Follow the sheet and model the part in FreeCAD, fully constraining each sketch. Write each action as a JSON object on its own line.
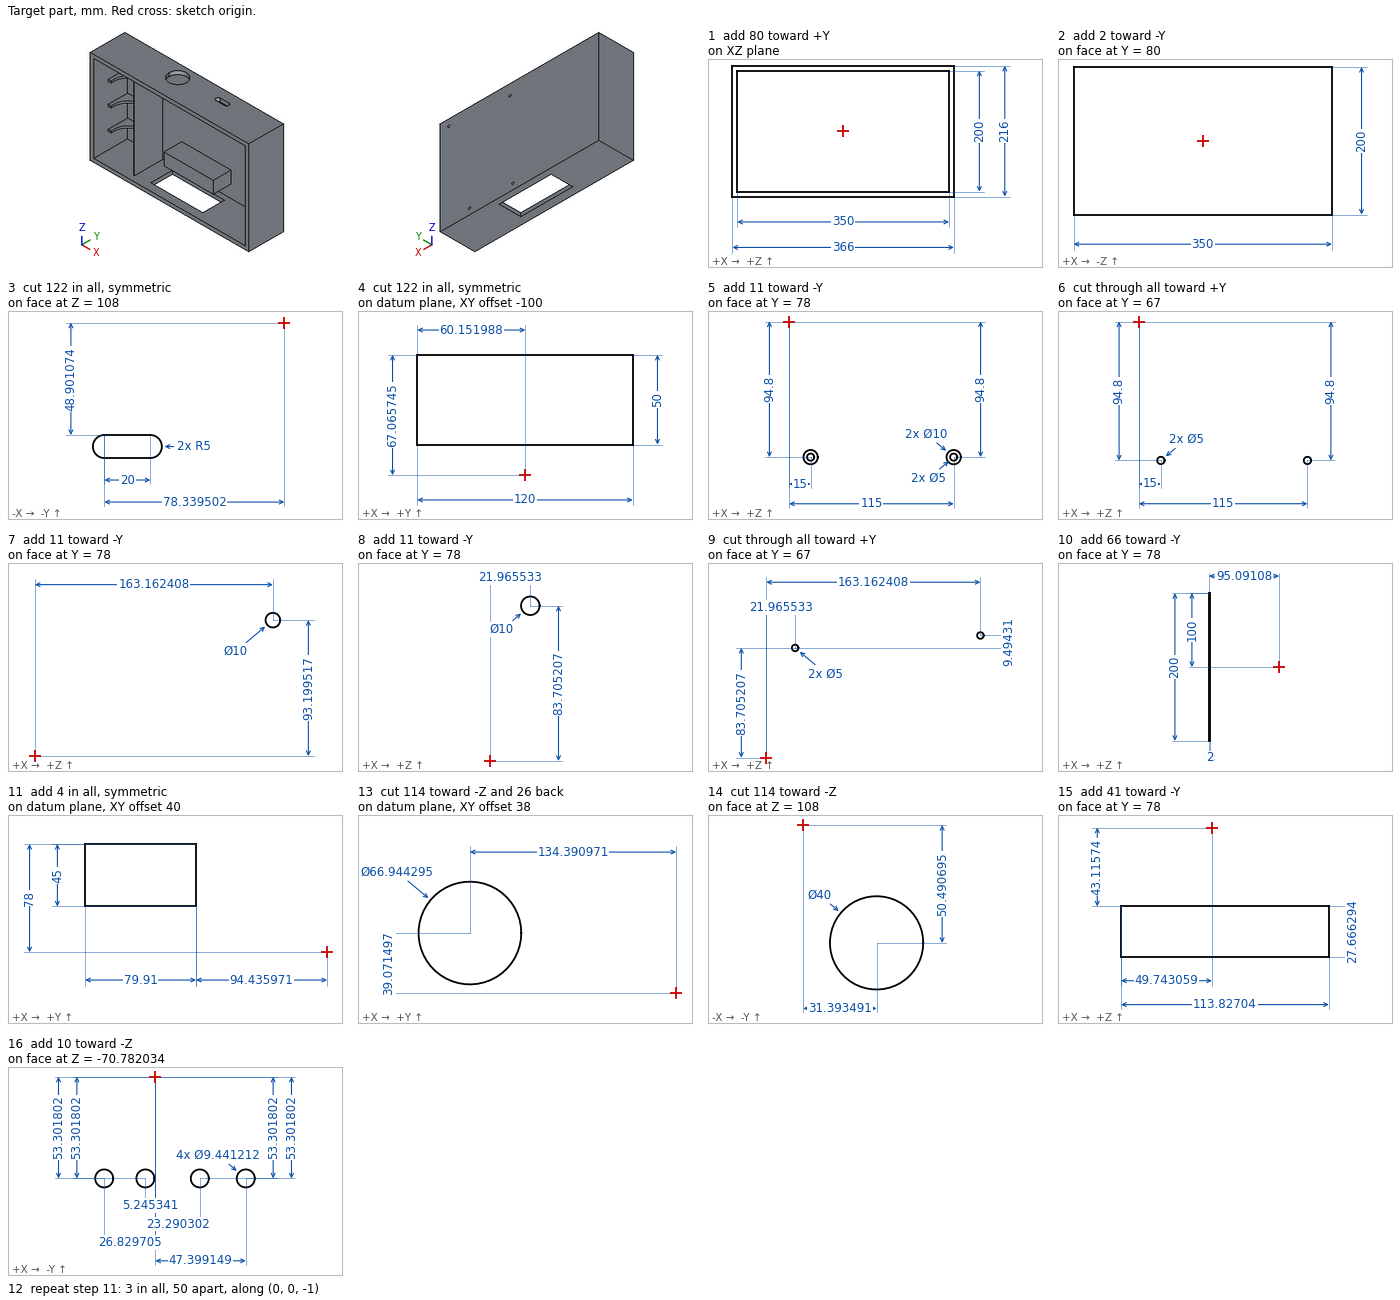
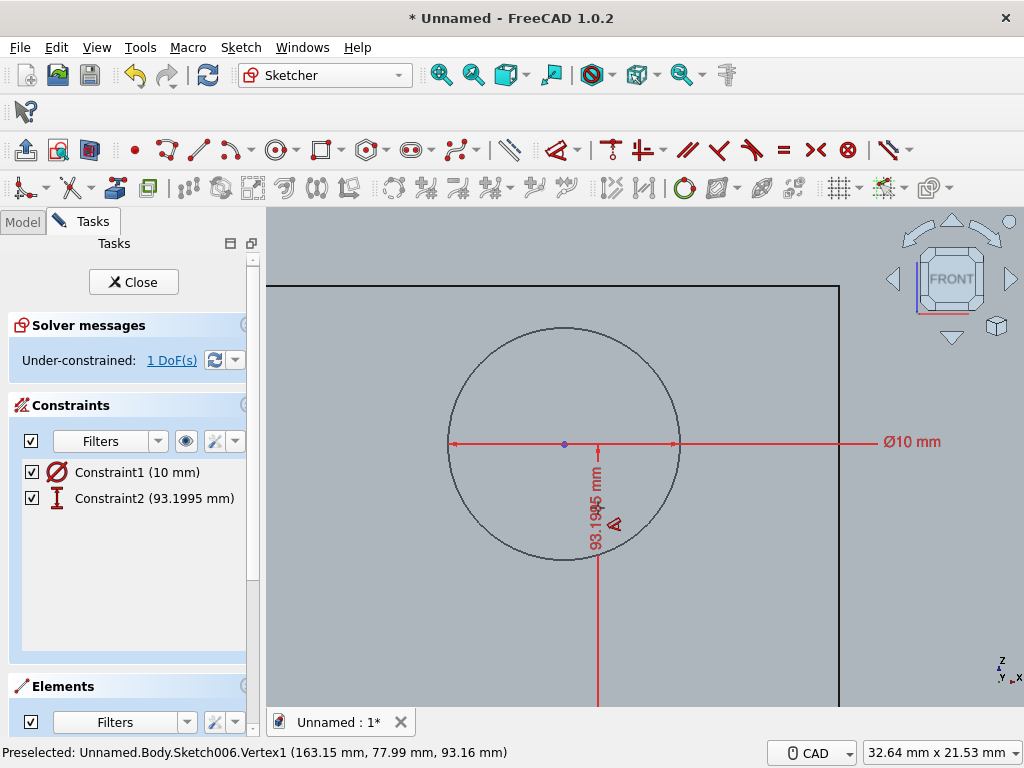
{"action": "left_click", "coordinate": [564, 444]}
{"action": "left_click", "coordinate": [429, 410]}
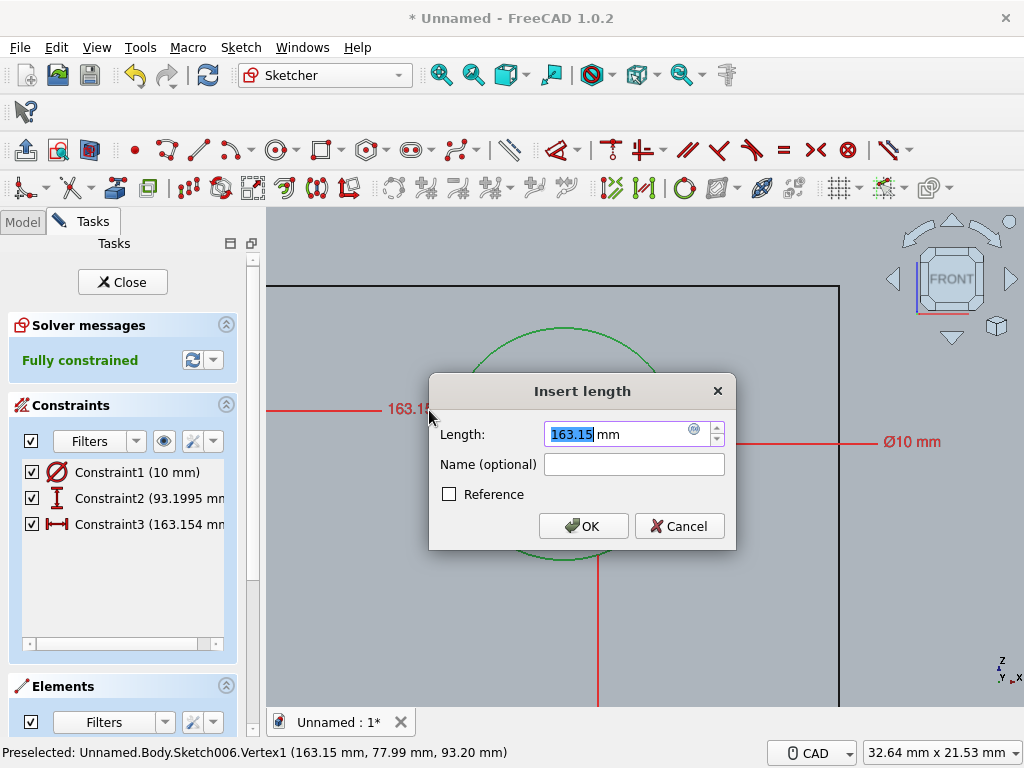
{"action": "type", "text": "163.162408"}
{"action": "key", "text": "Return"}
{"action": "key", "text": "Escape"}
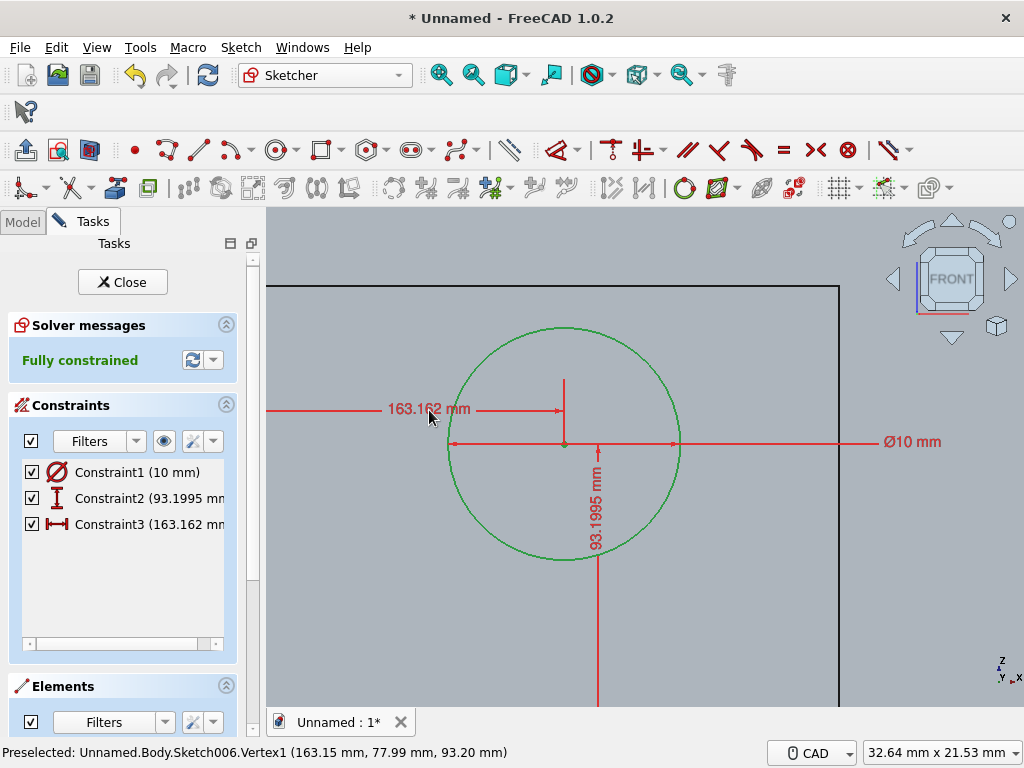
{"action": "left_click", "coordinate": [123, 282]}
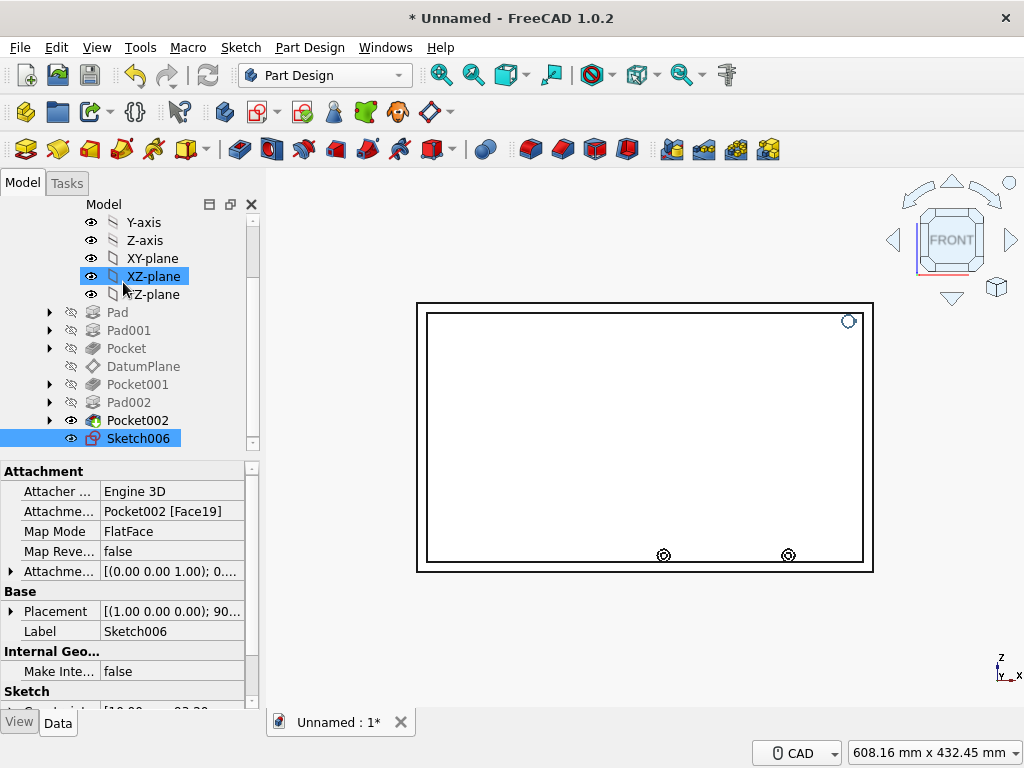
{"action": "left_click", "coordinate": [26, 150]}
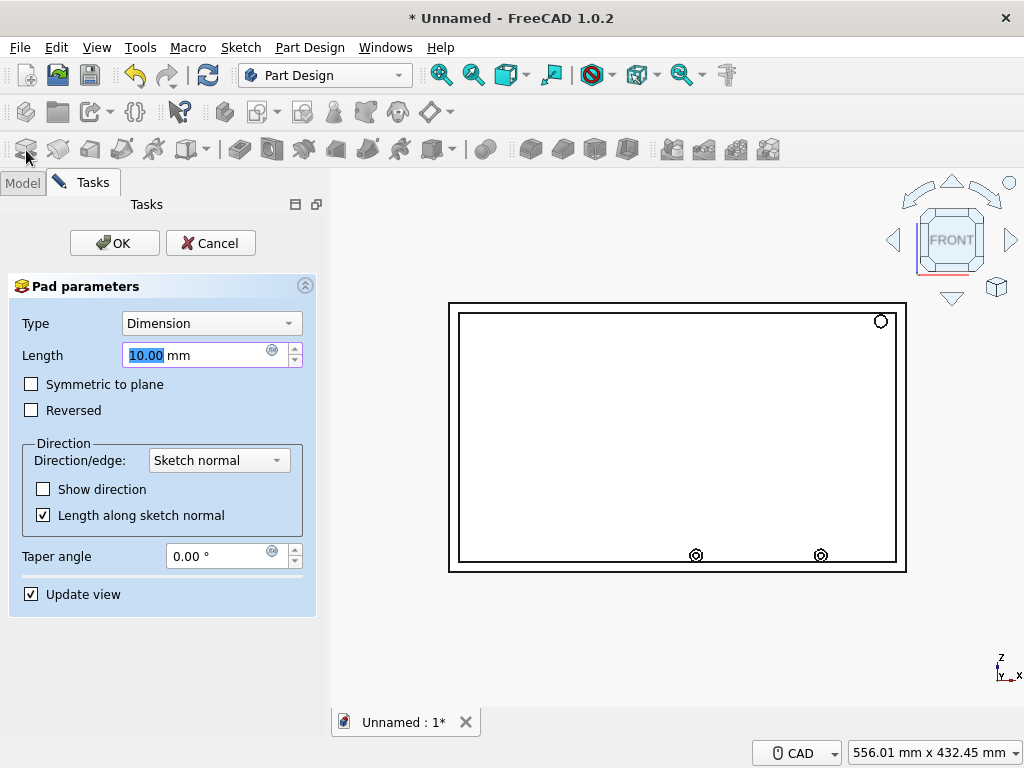
{"action": "type", "text": "11"}
{"action": "key", "text": "Tab"}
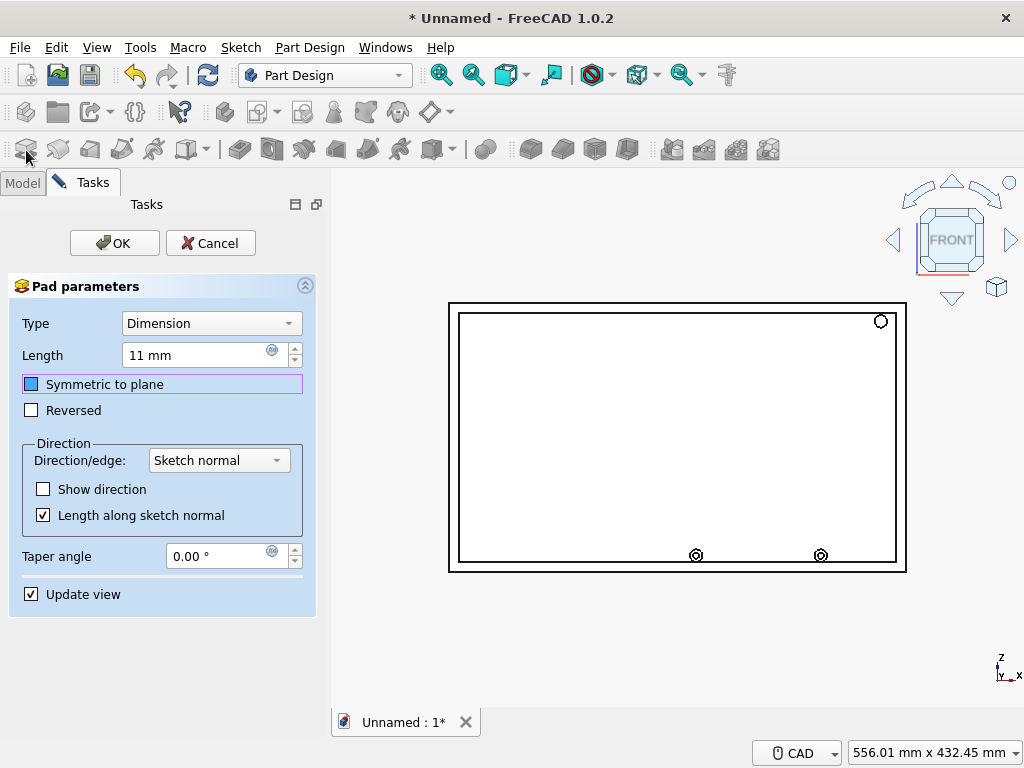
{"action": "left_click", "coordinate": [115, 243]}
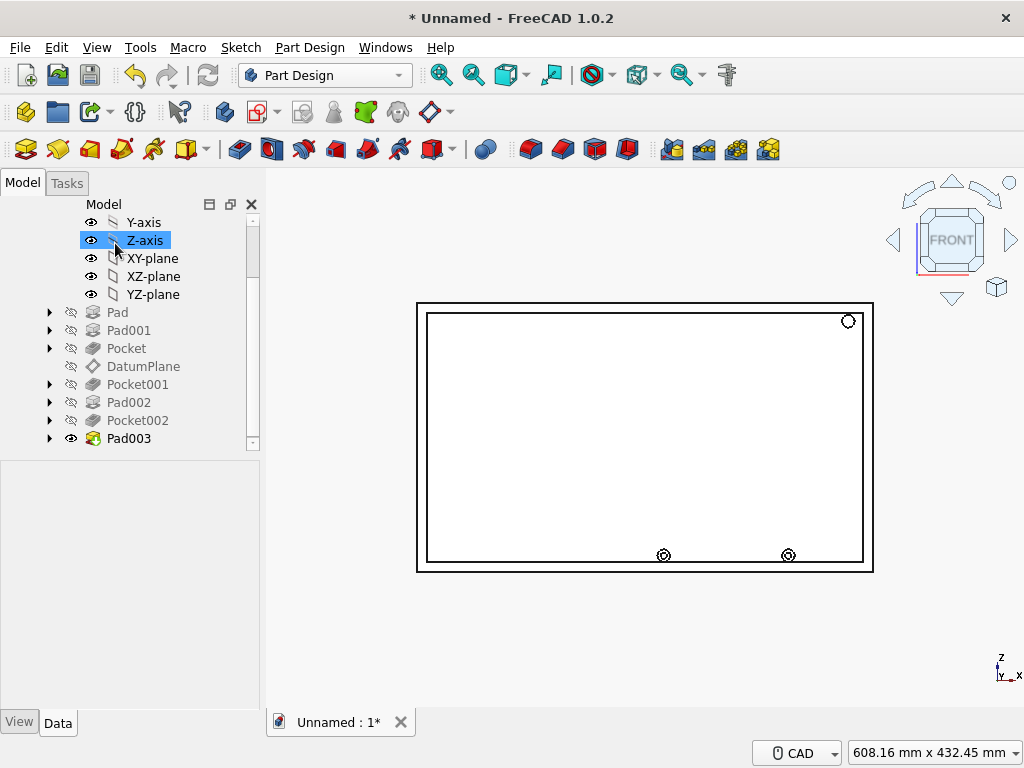
{"action": "left_click", "coordinate": [583, 437]}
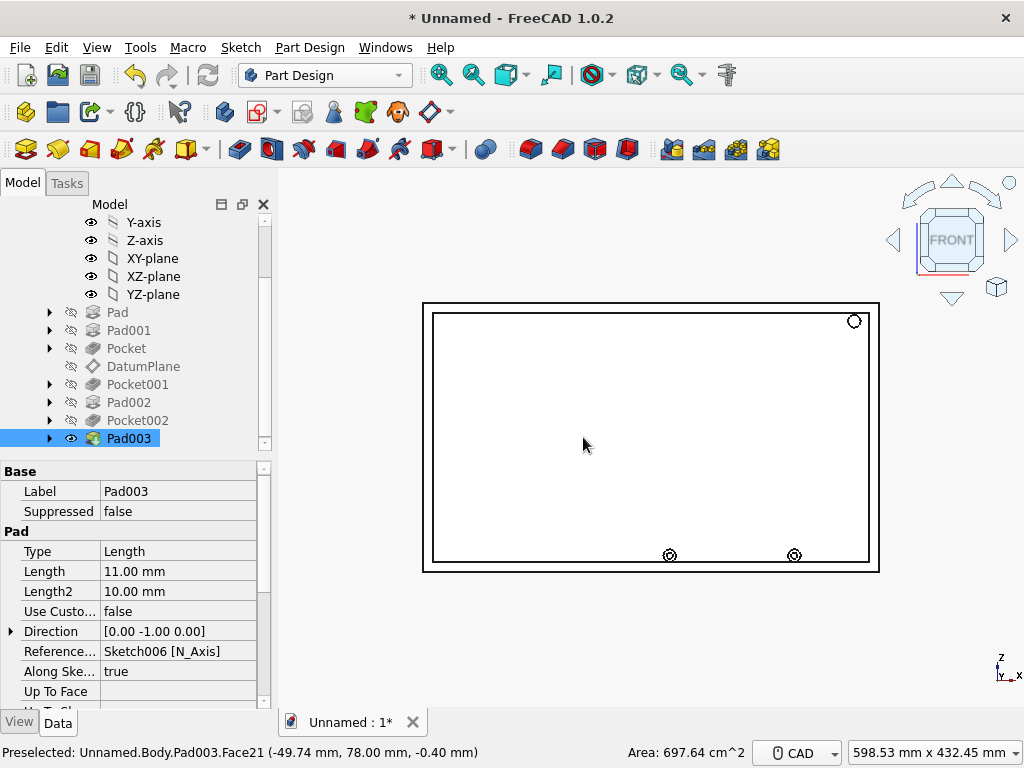
{"action": "left_click", "coordinate": [258, 112]}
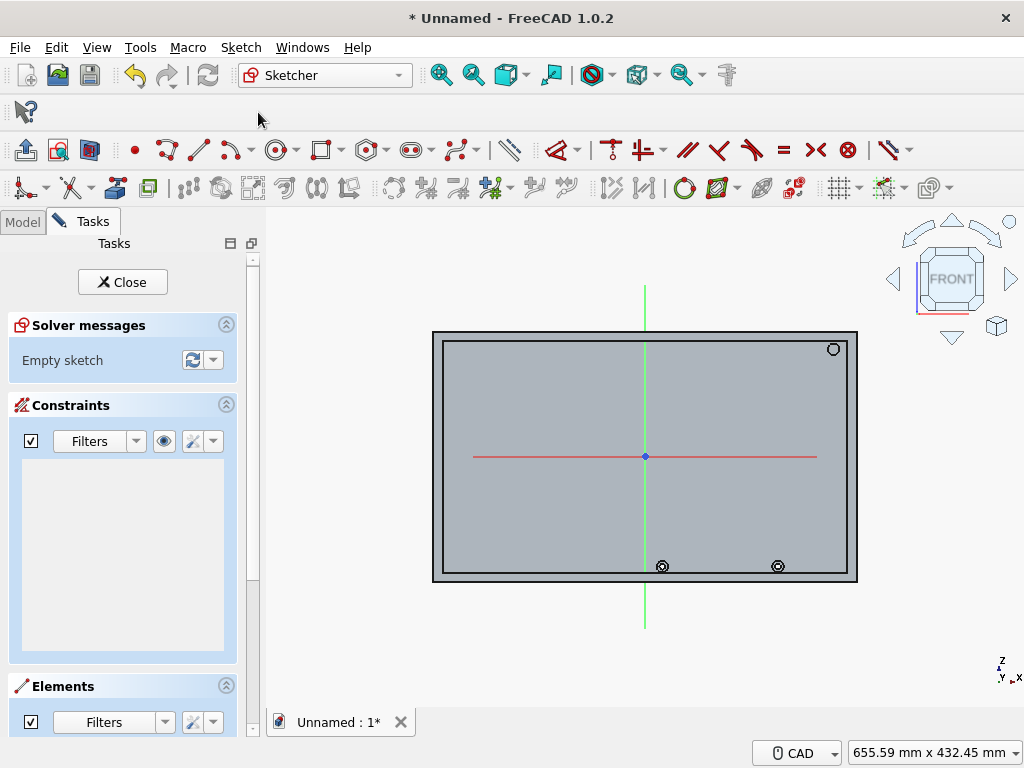
{"action": "key", "text": "q s"}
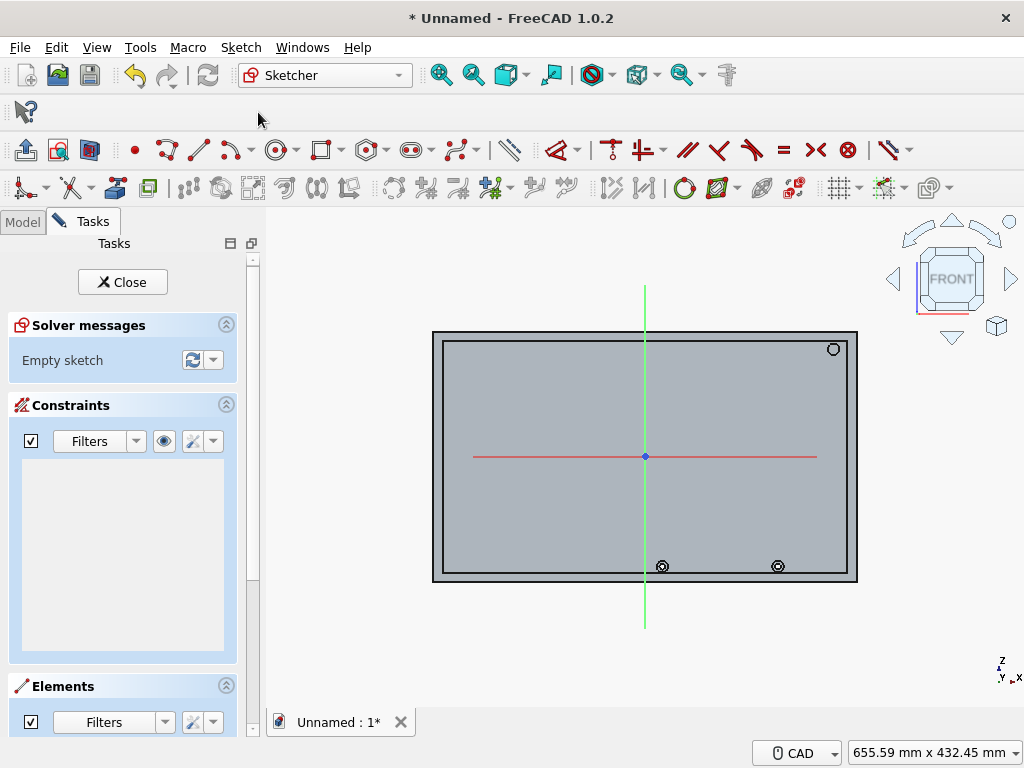
{"action": "scroll", "coordinate": [675, 355], "scroll_direction": "up", "scroll_amount": 15}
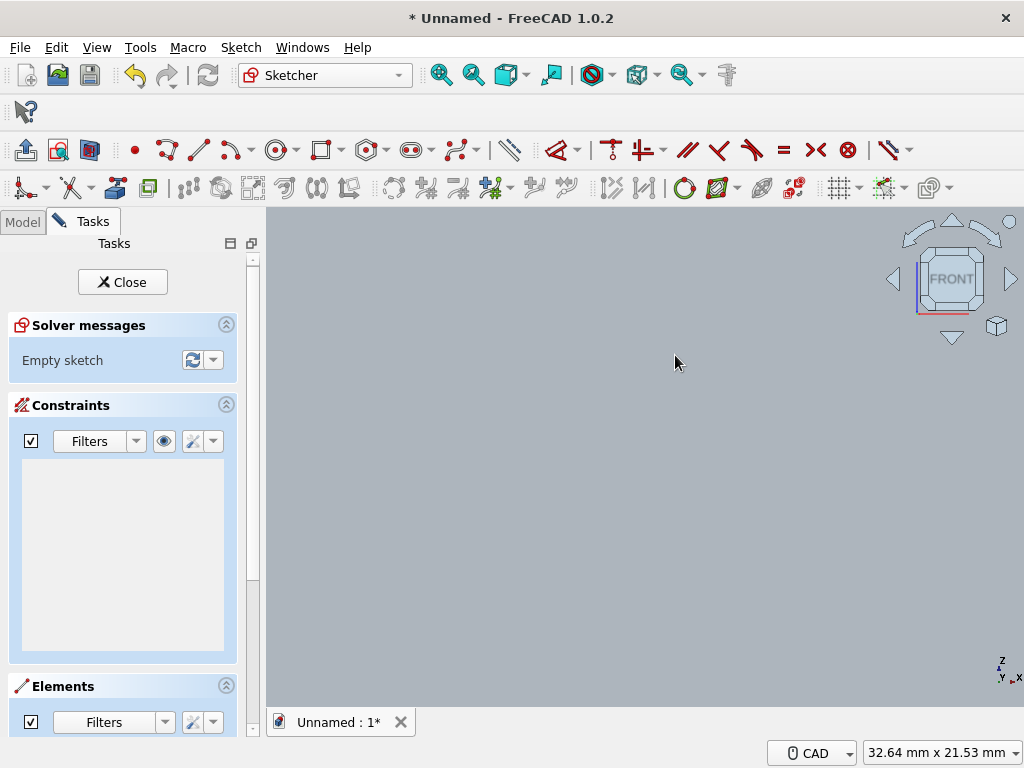
{"action": "key", "text": "g c"}